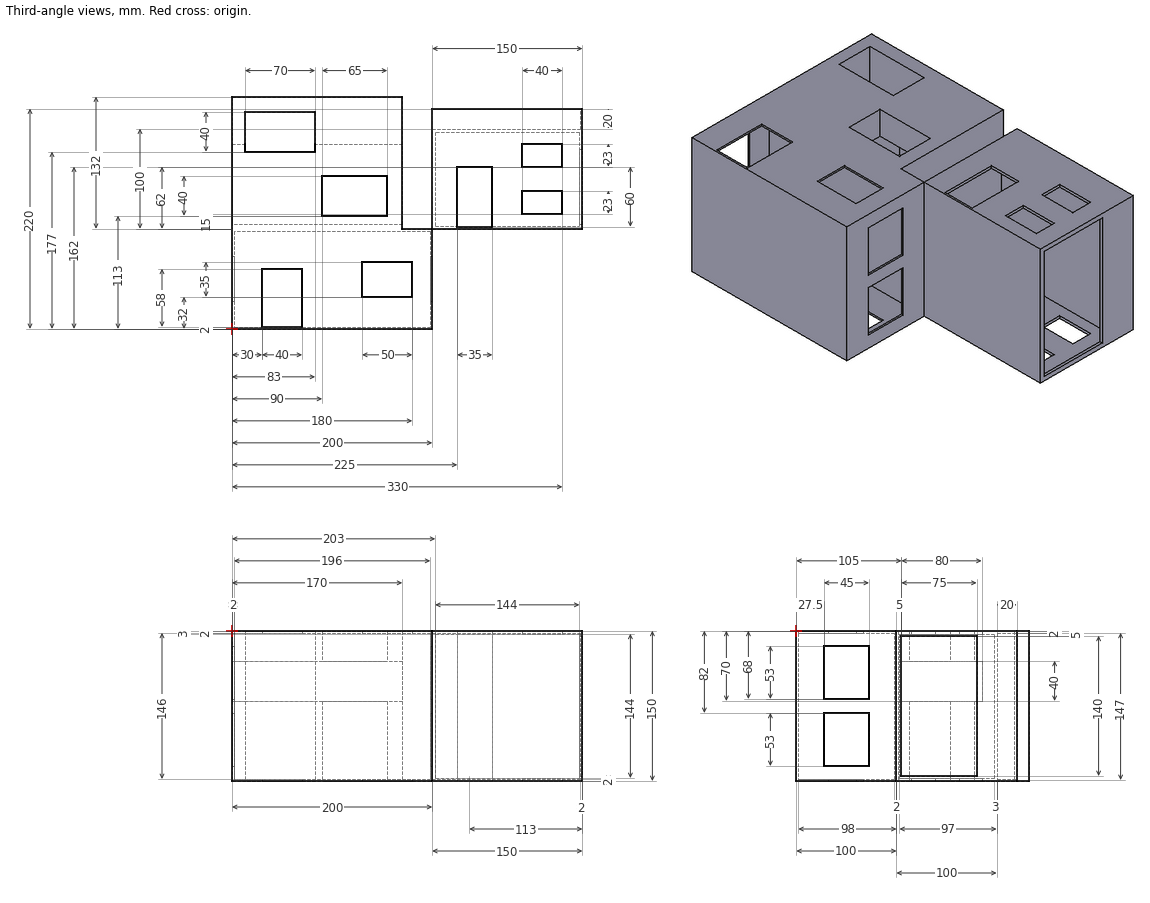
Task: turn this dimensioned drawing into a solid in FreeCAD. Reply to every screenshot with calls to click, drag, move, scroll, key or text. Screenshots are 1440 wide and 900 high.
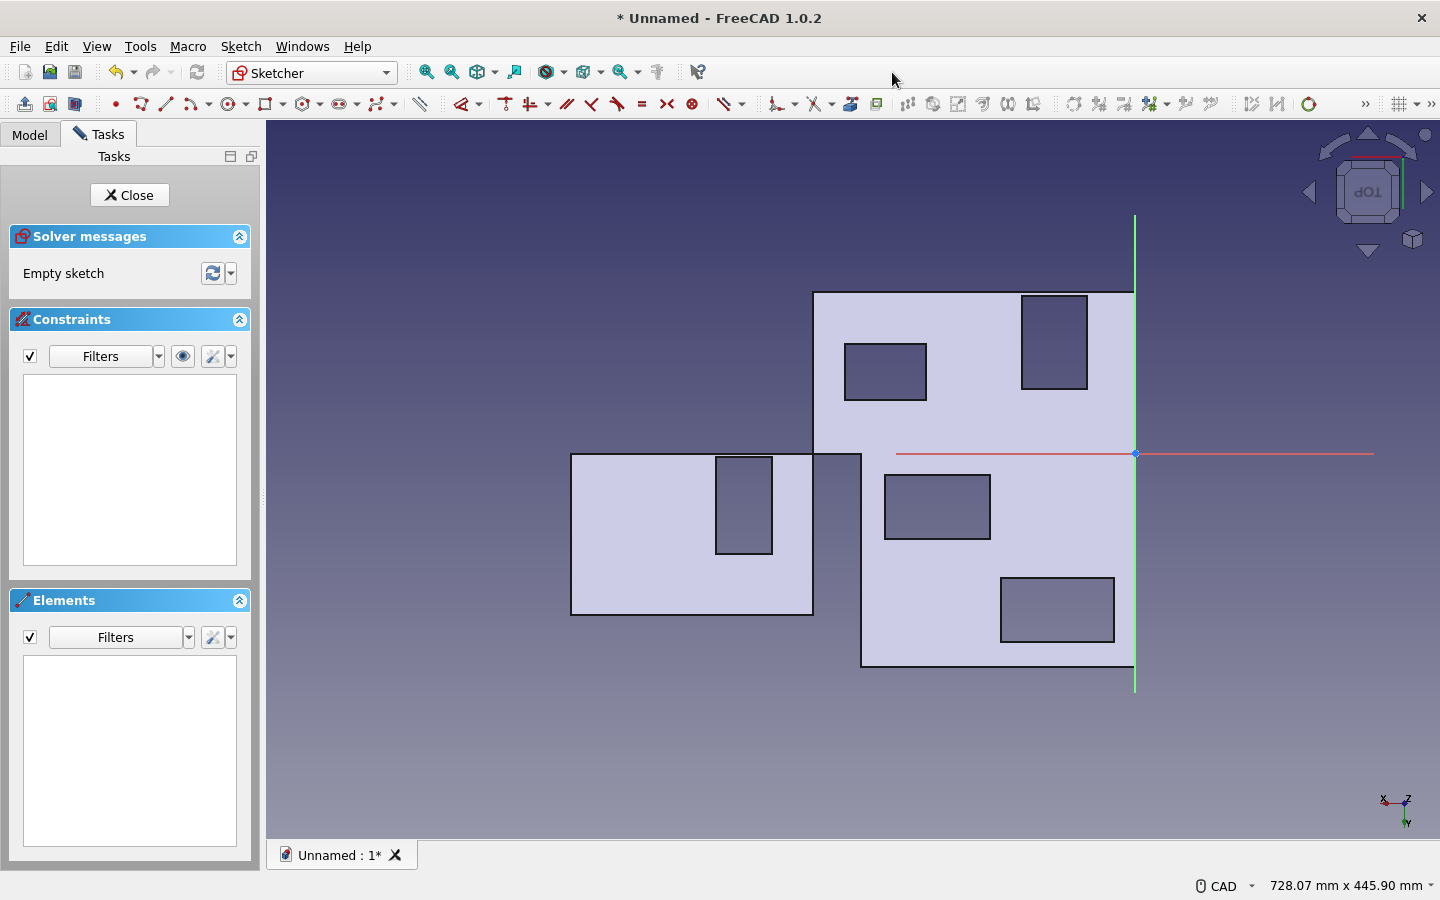
scroll(586, 552, up, 7)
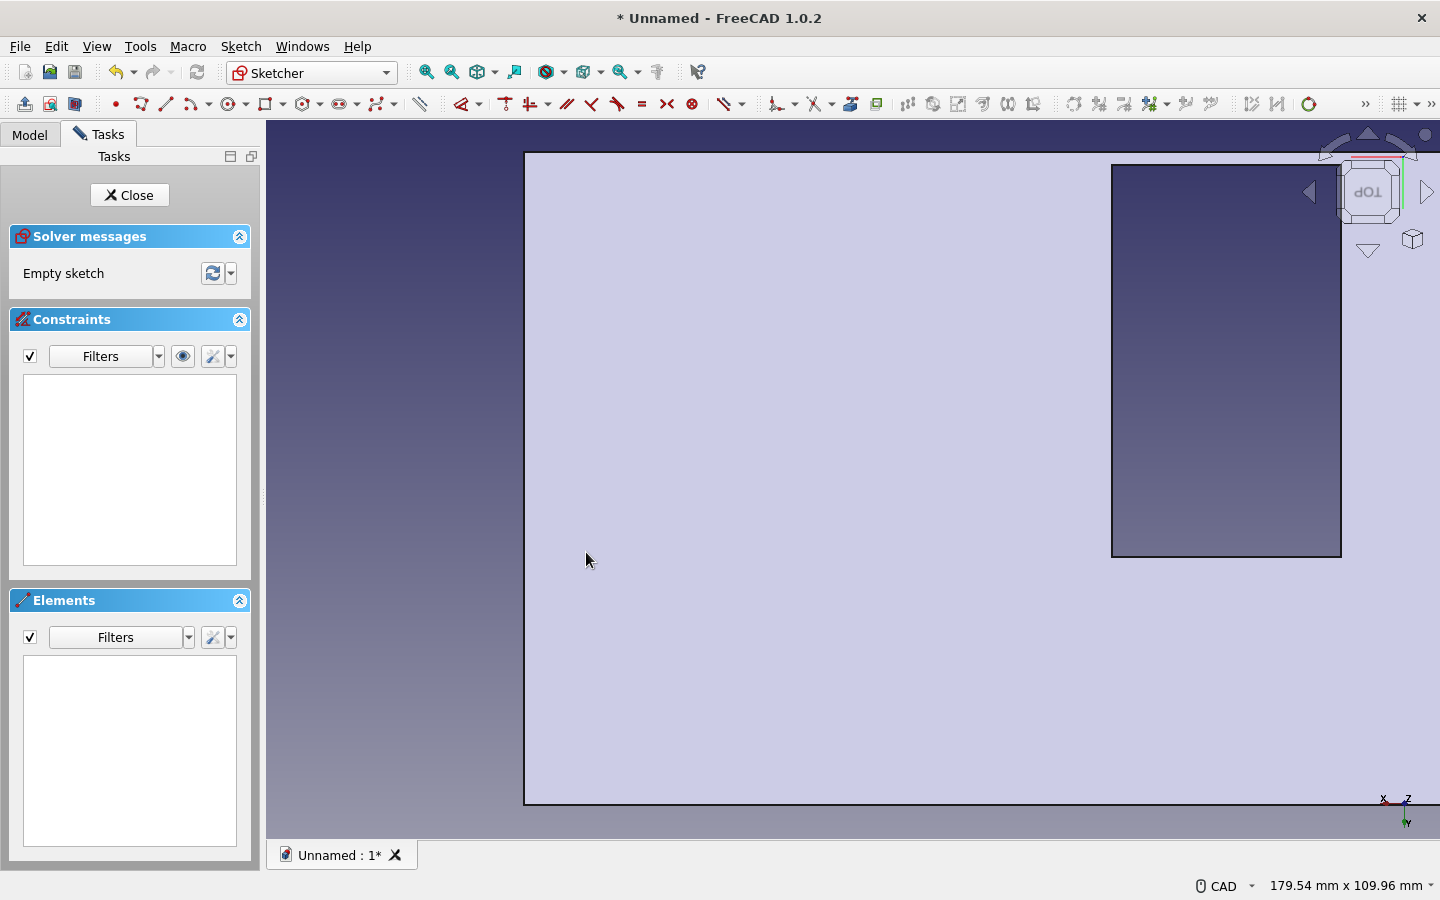
click(264, 104)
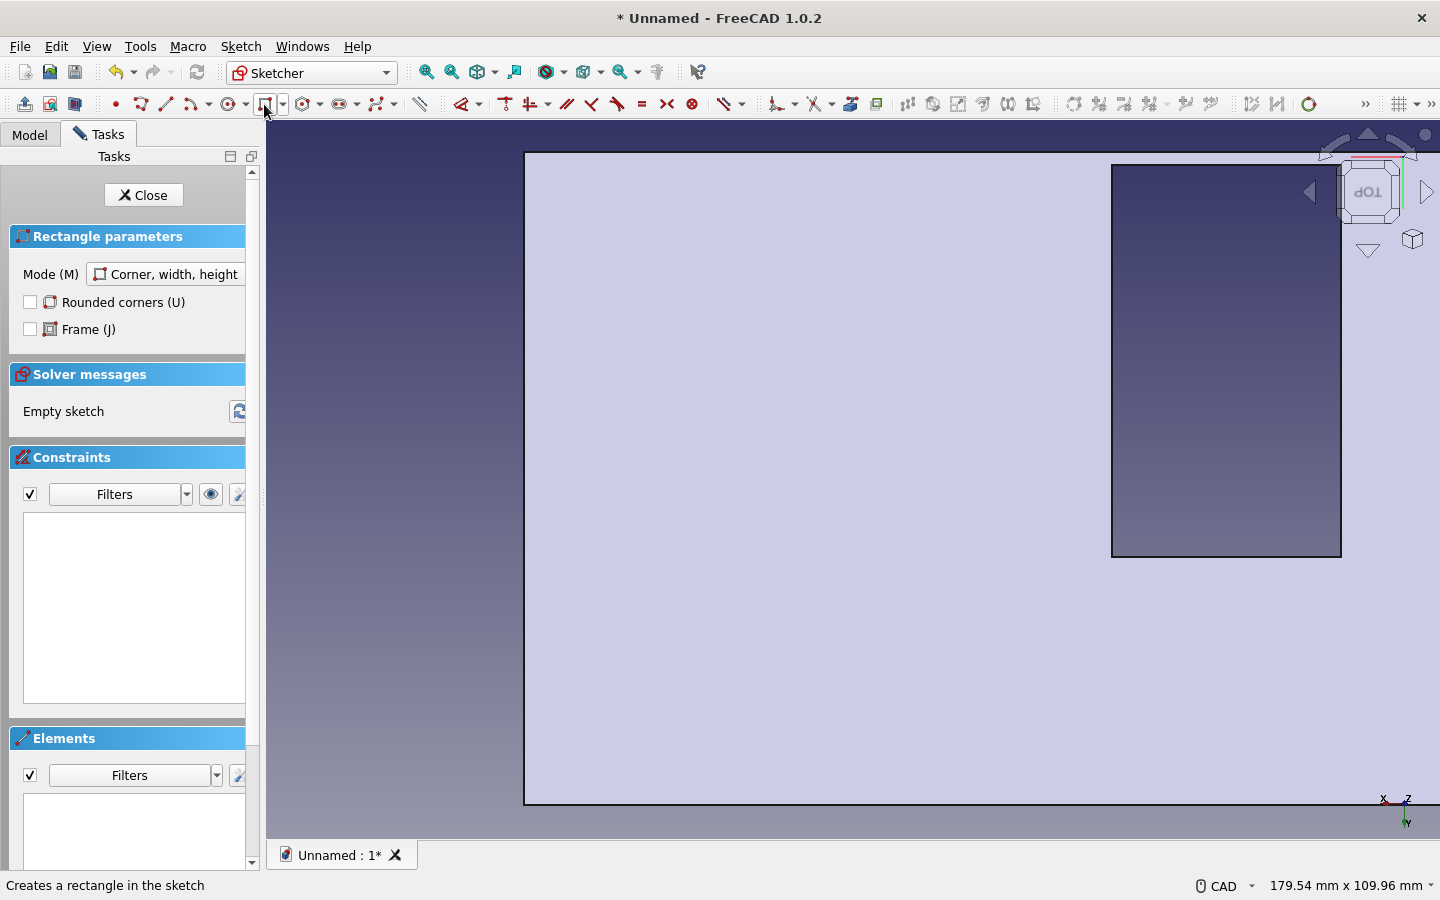
click(654, 250)
move(916, 400)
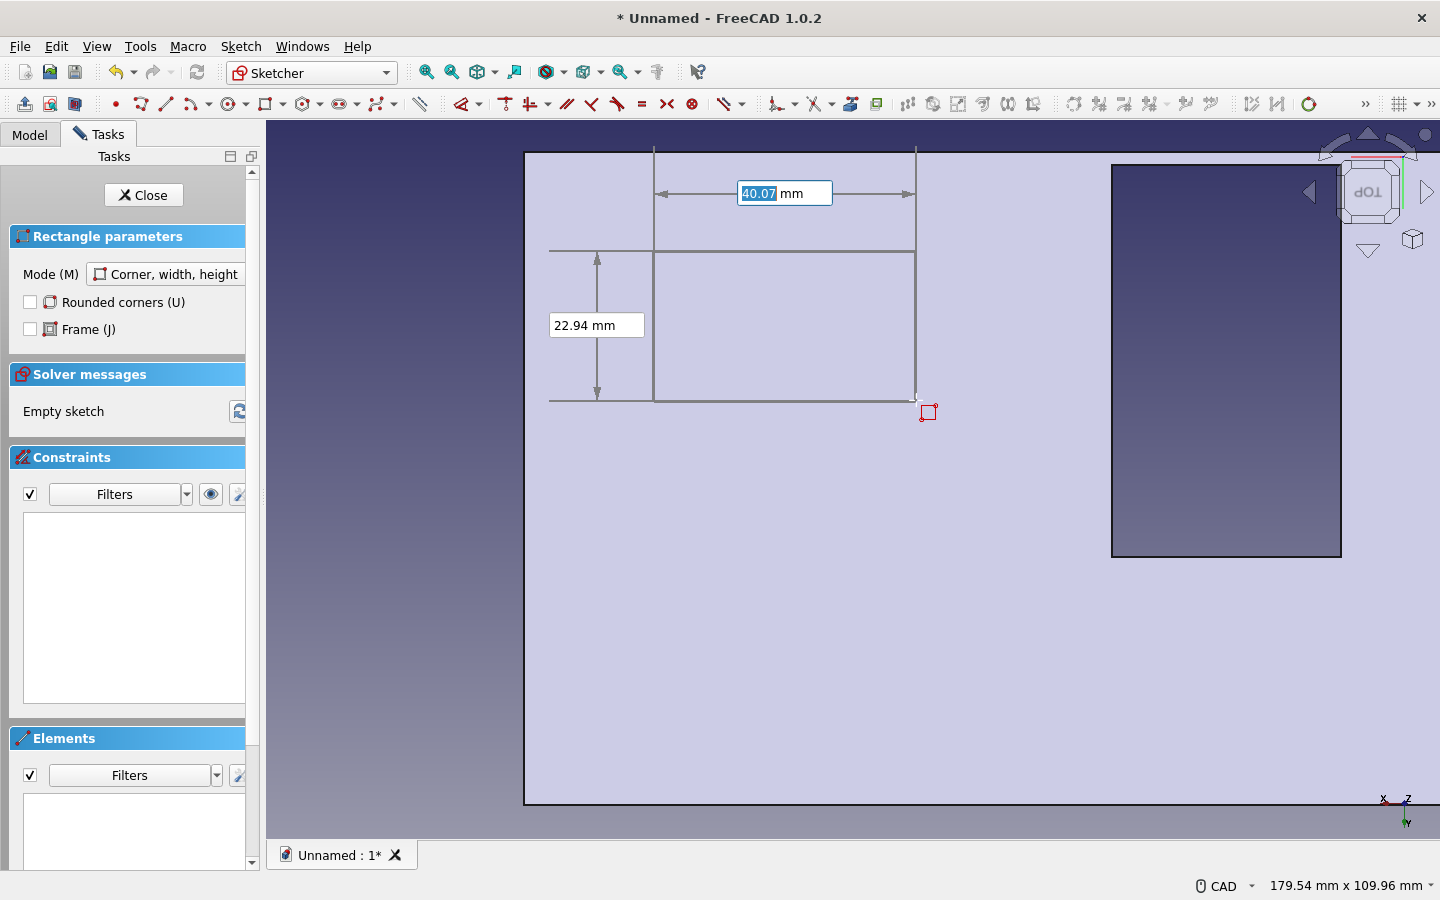
text(40)
key(Tab)
text(23)
key(Return)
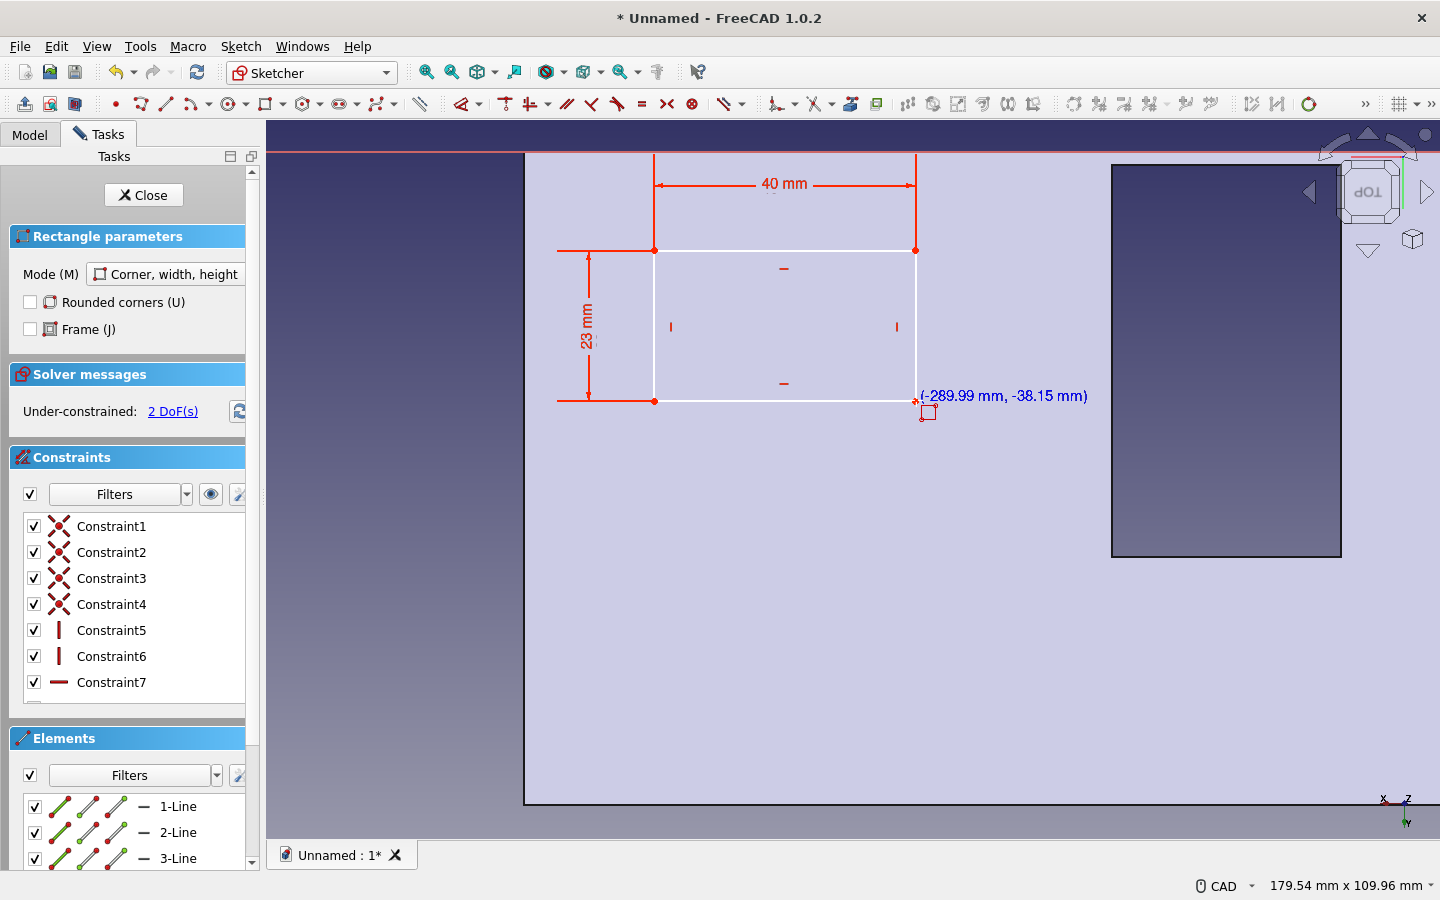
click(654, 557)
move(916, 707)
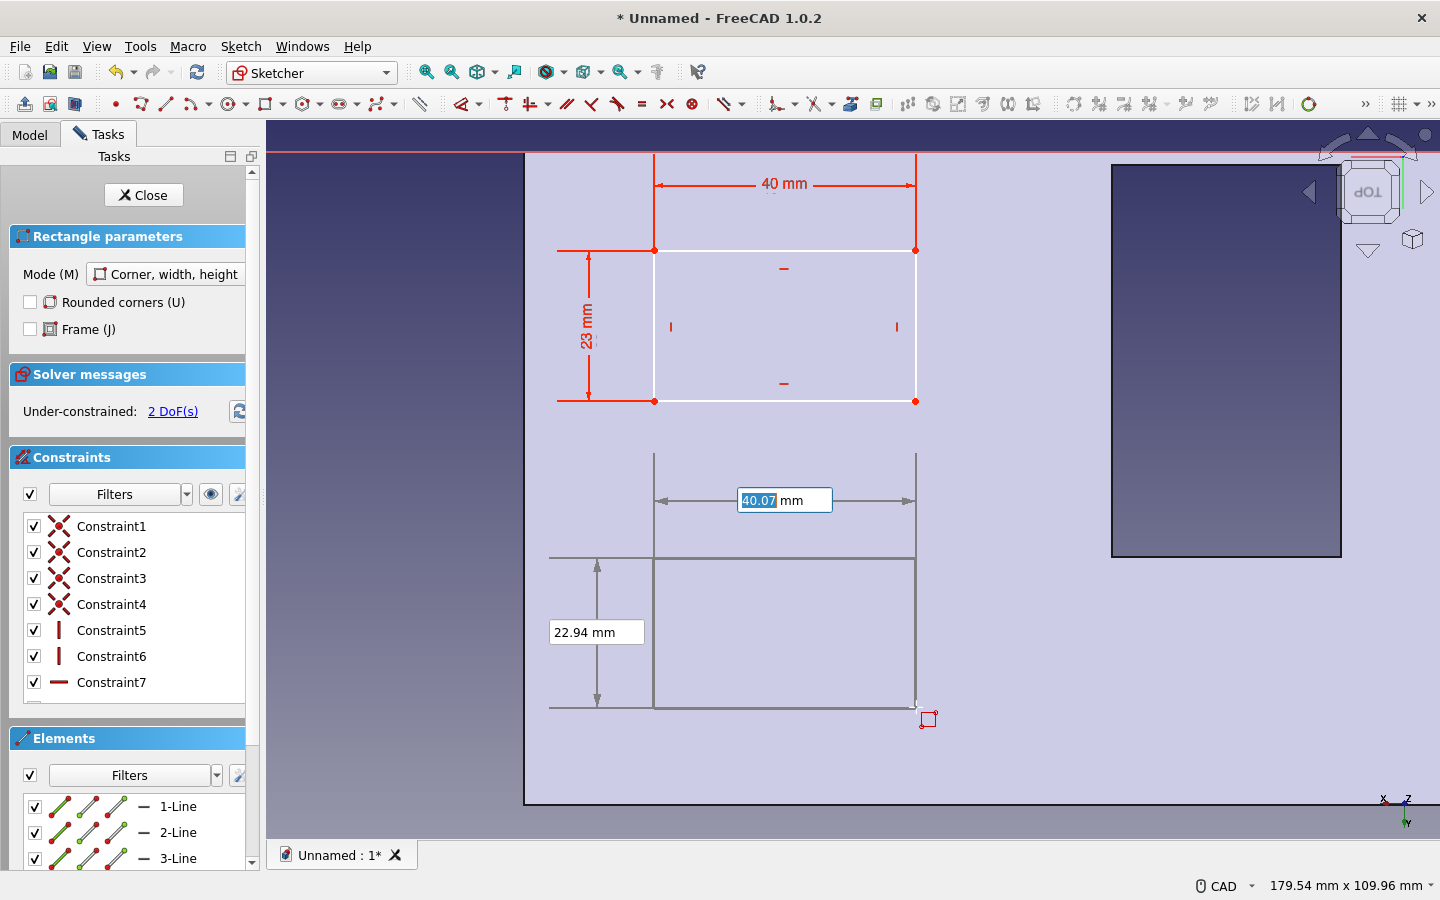
text(40)
key(Tab)
text(23)
key(Return)
key(Escape)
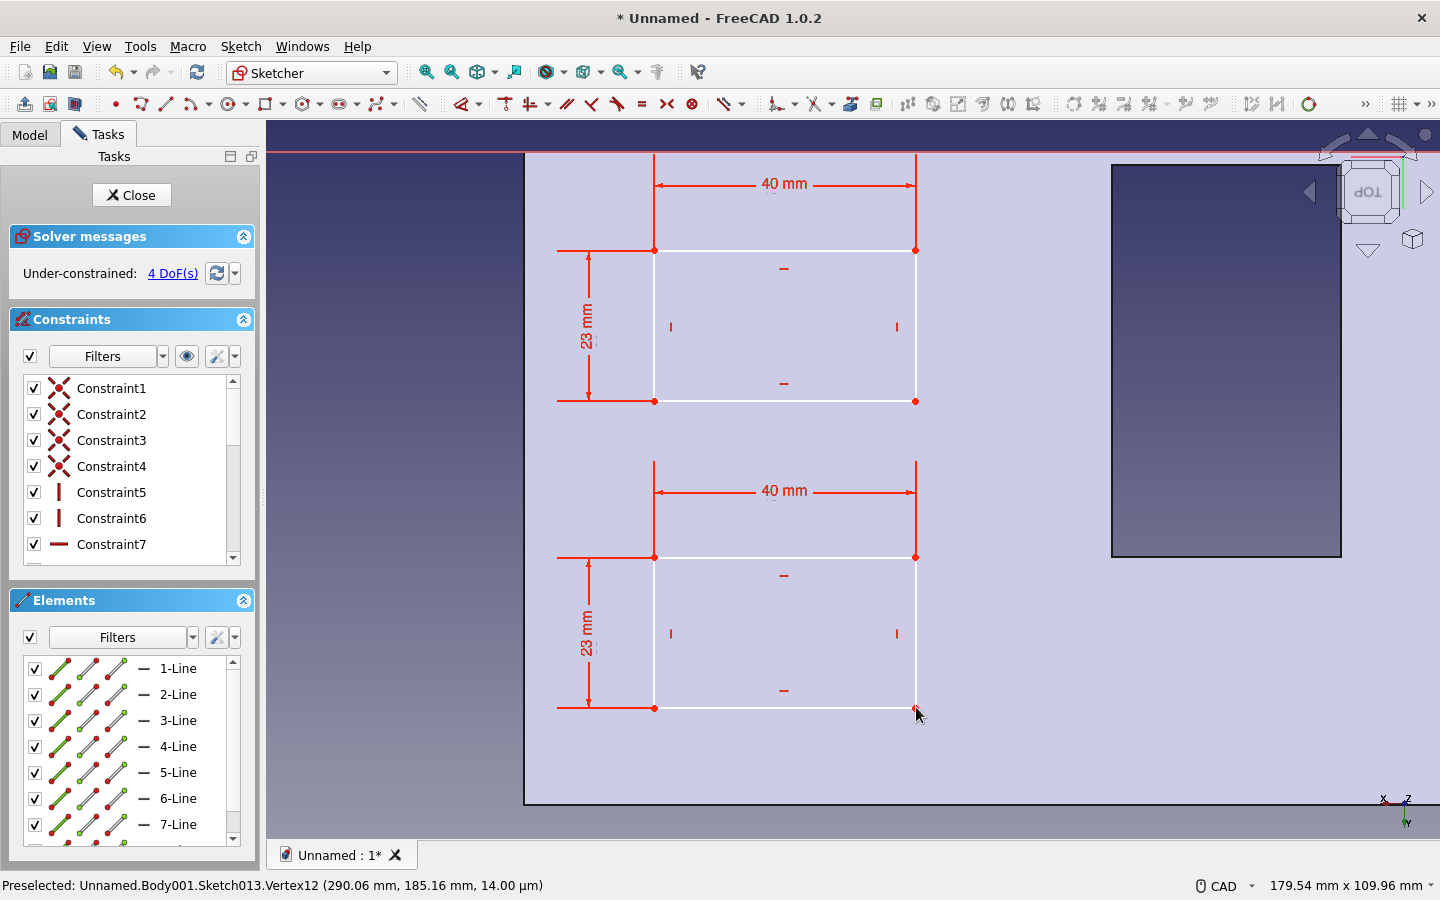
click(460, 104)